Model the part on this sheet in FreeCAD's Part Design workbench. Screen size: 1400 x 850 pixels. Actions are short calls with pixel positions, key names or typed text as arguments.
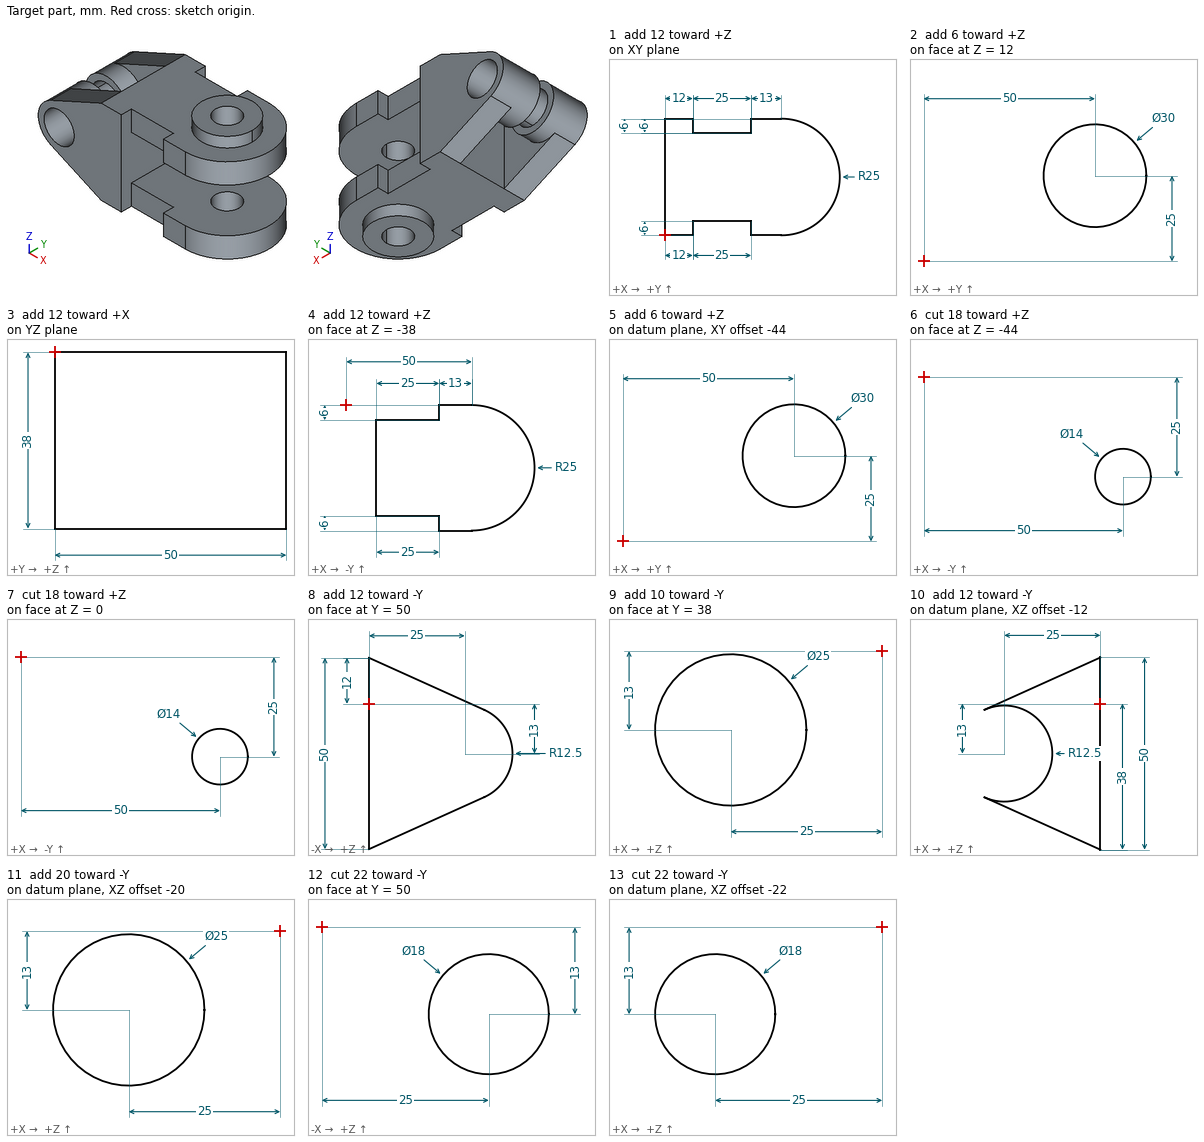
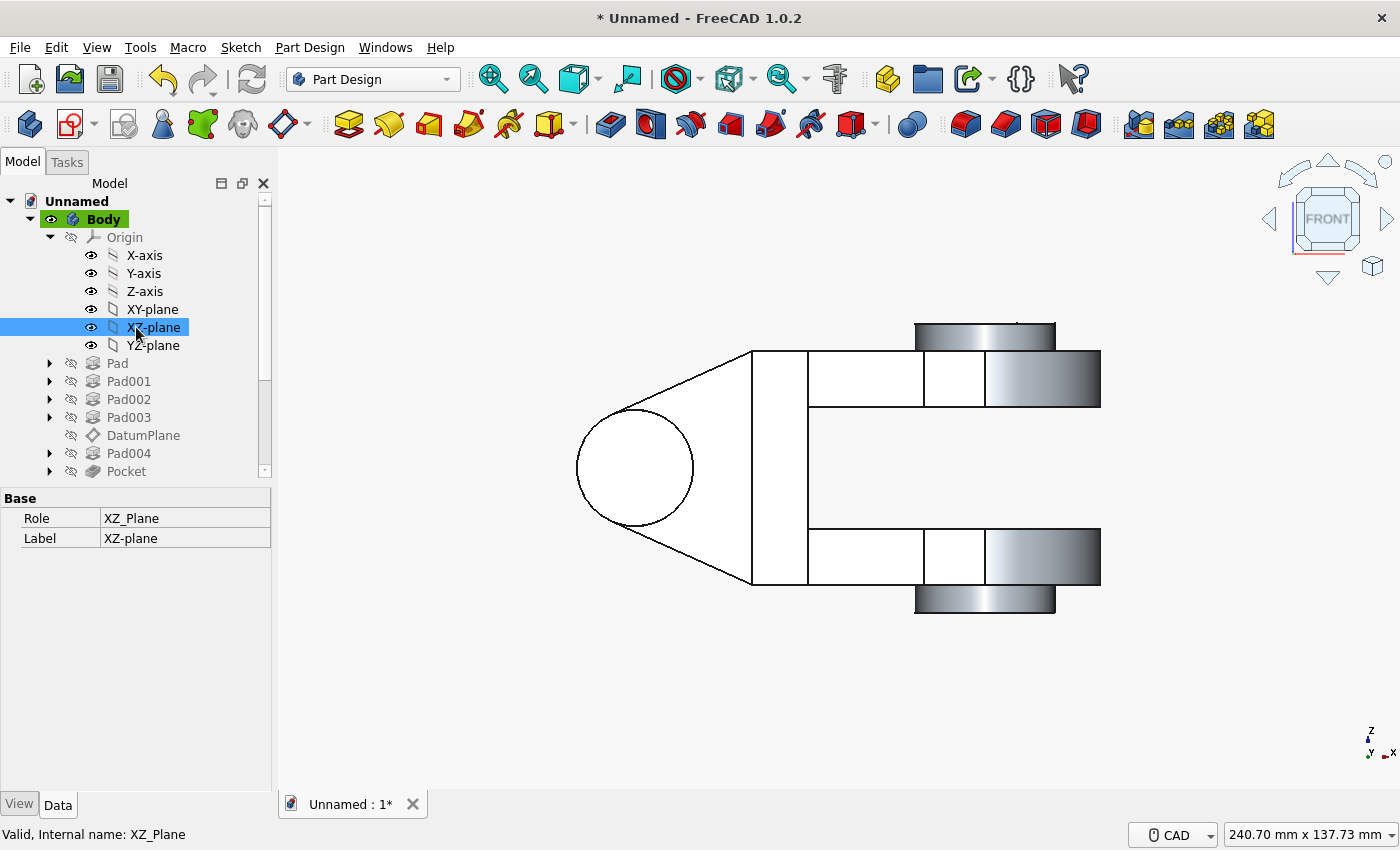
click(284, 124)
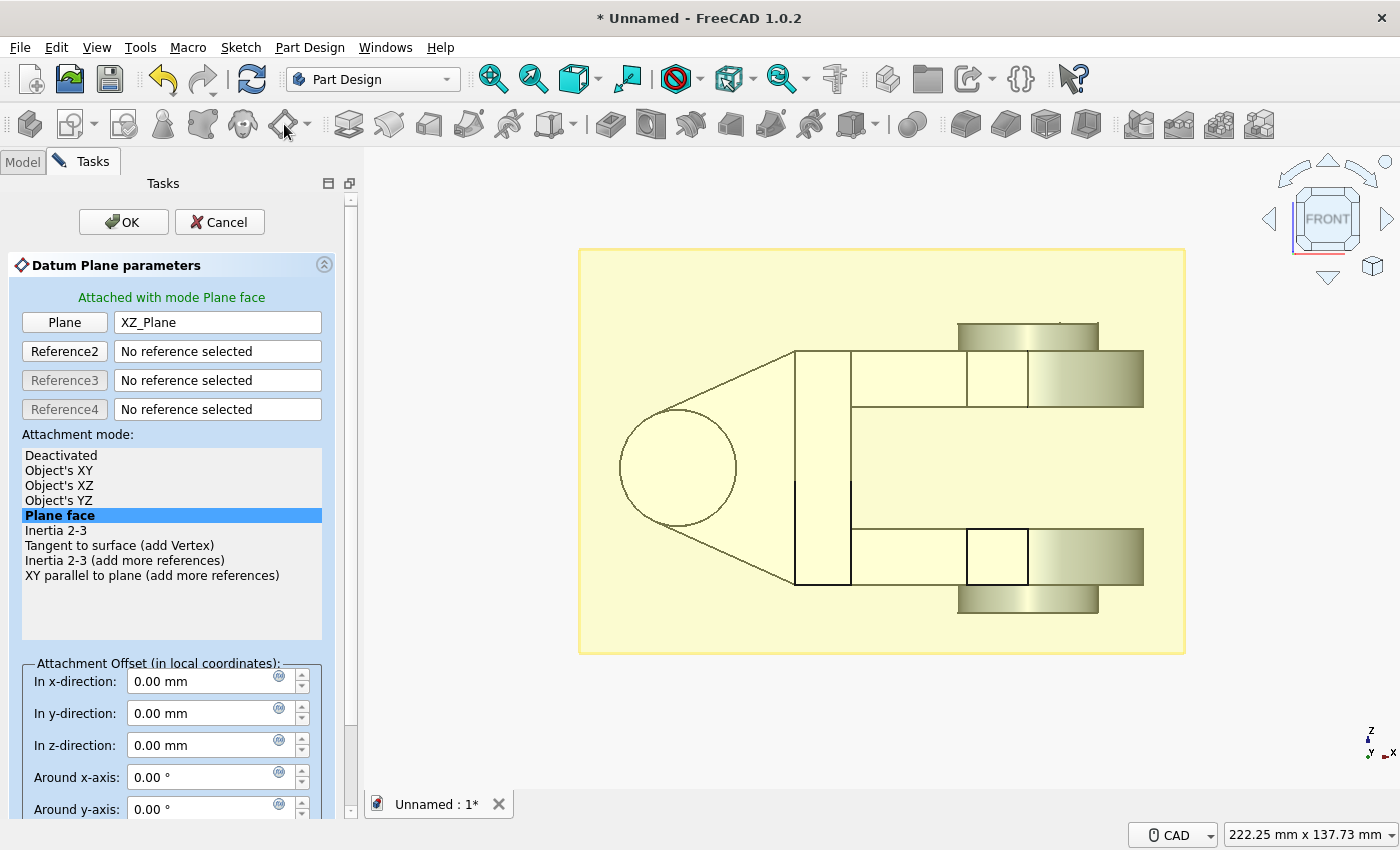
triple_click(210, 745)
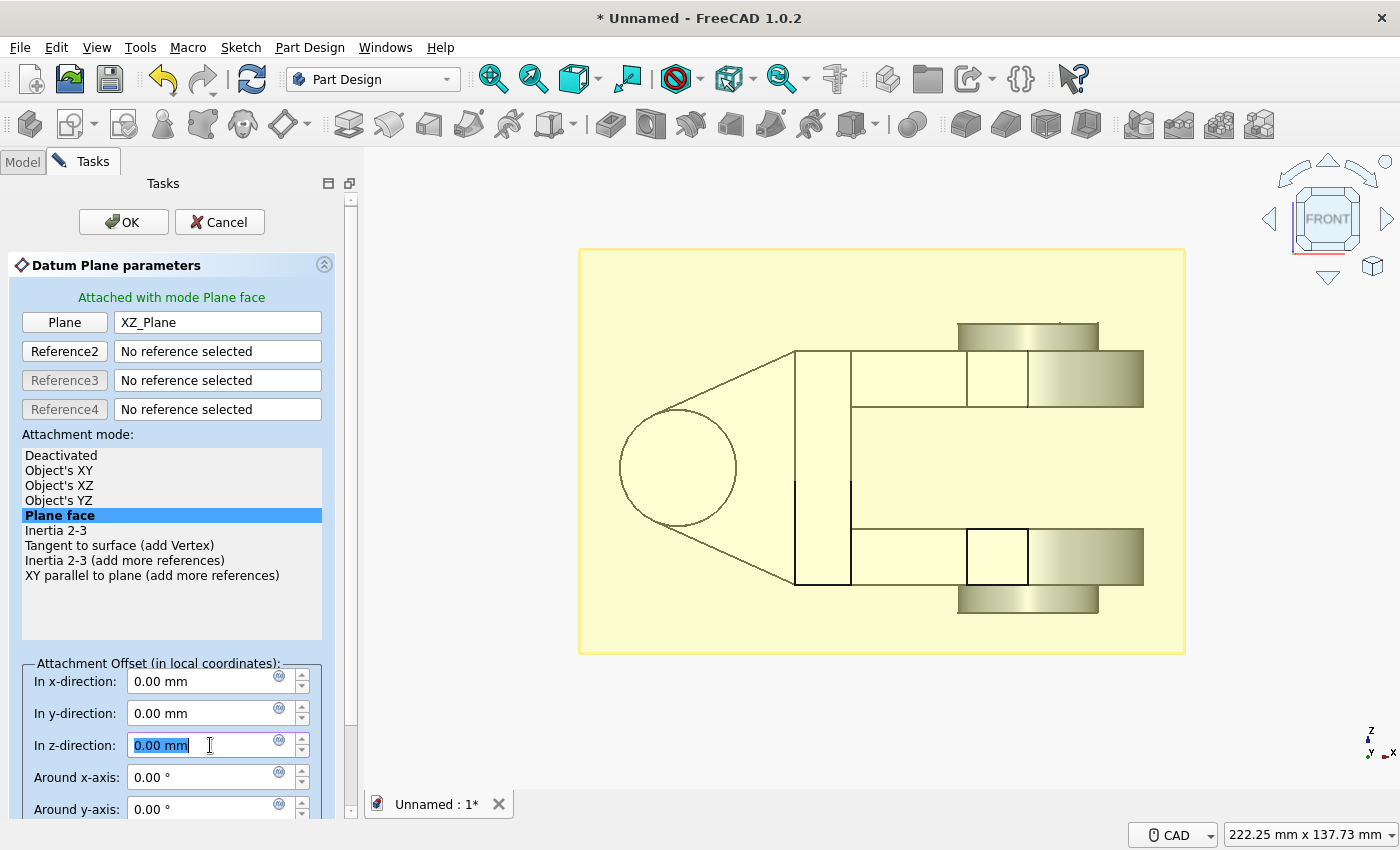
text(-12)
key(Tab)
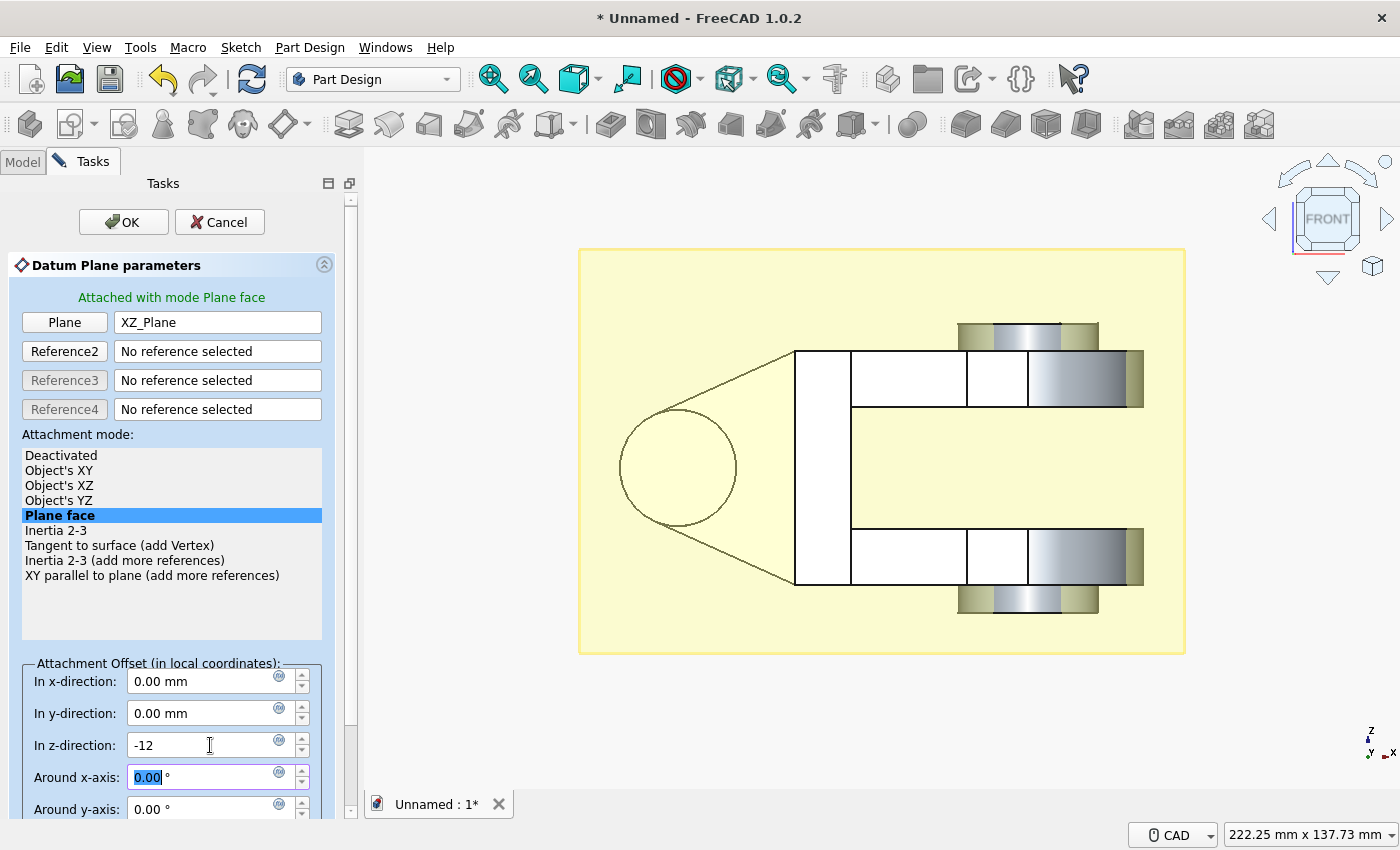
click(124, 222)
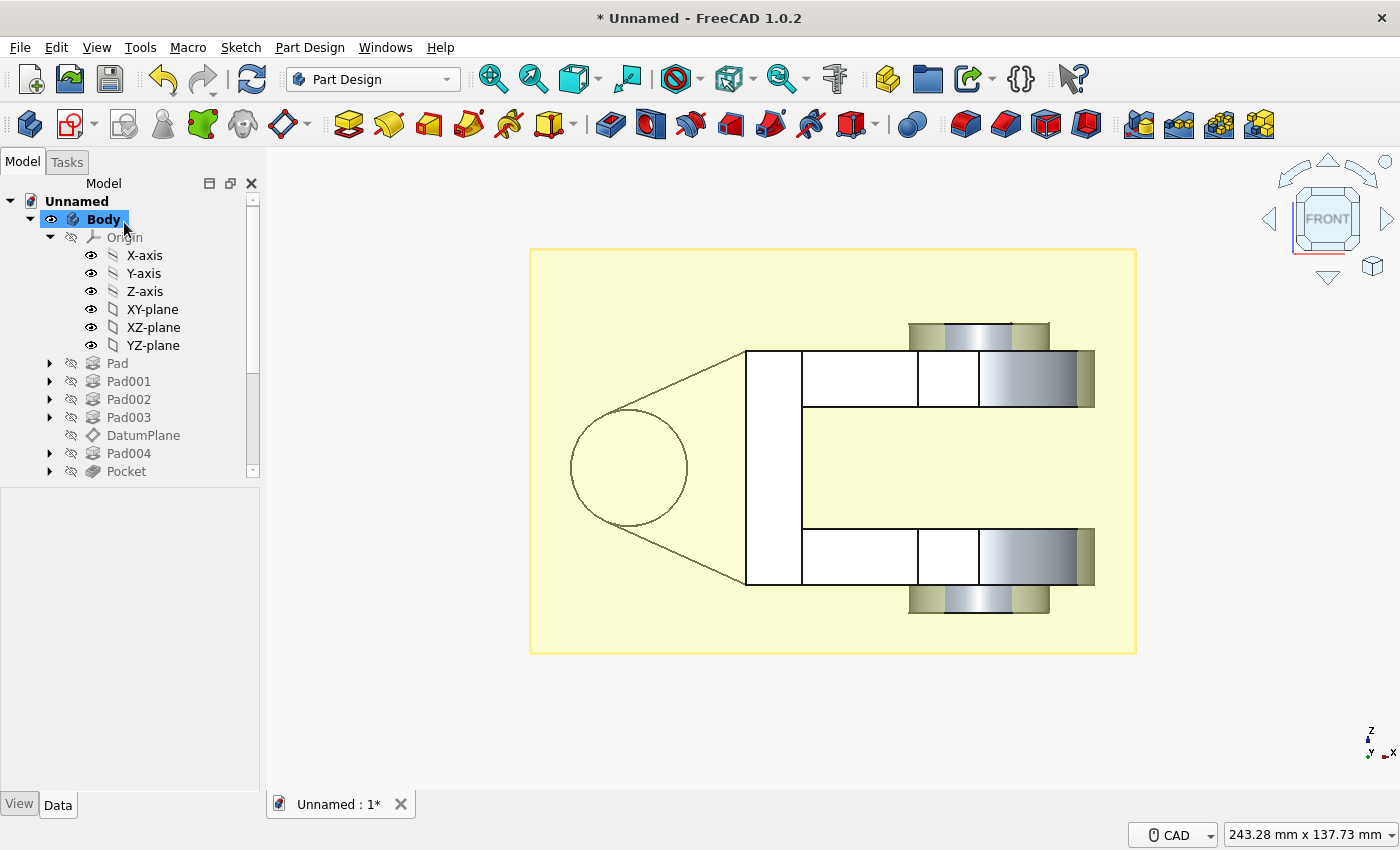
scroll(100, 341, down, 3)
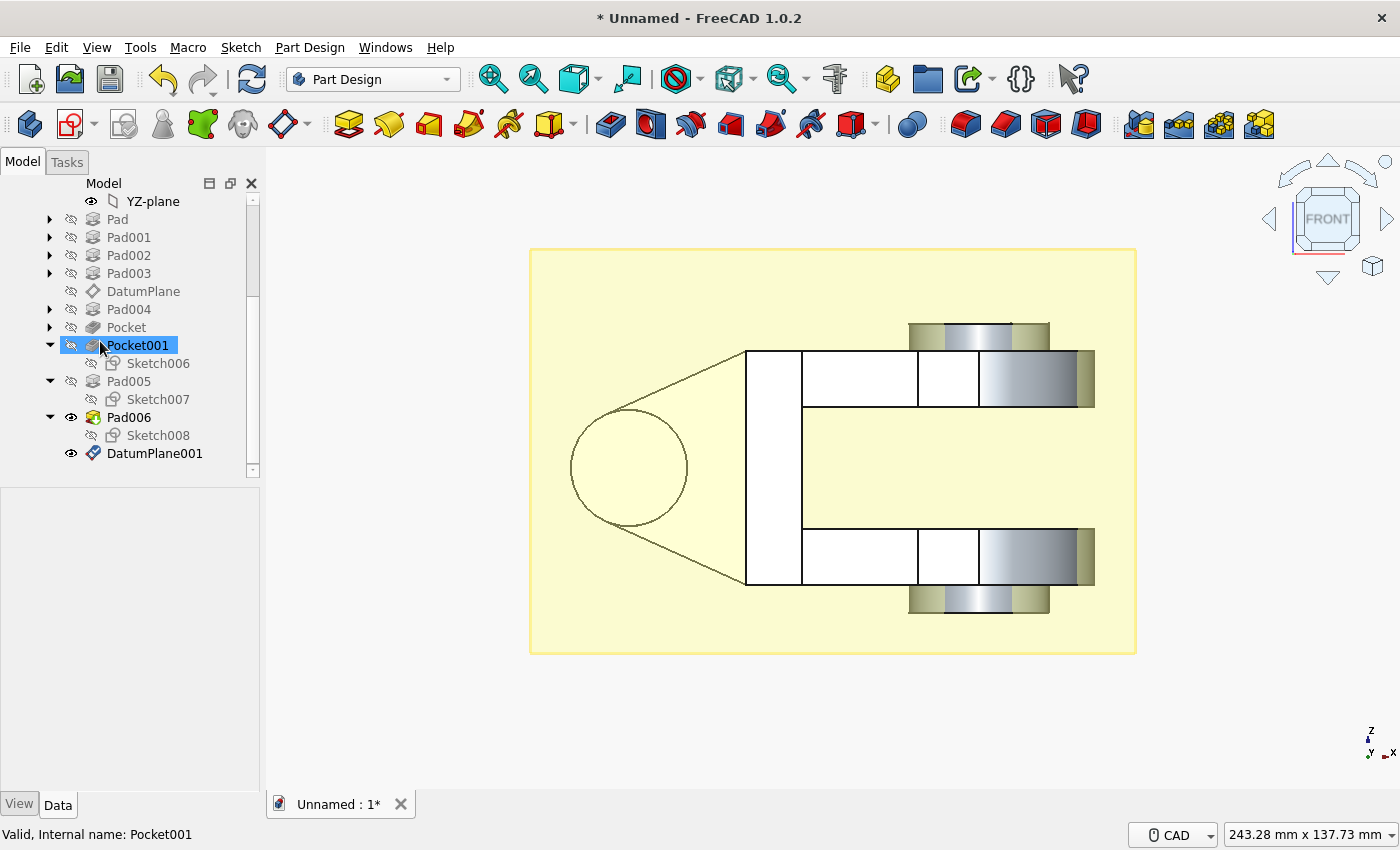
click(116, 453)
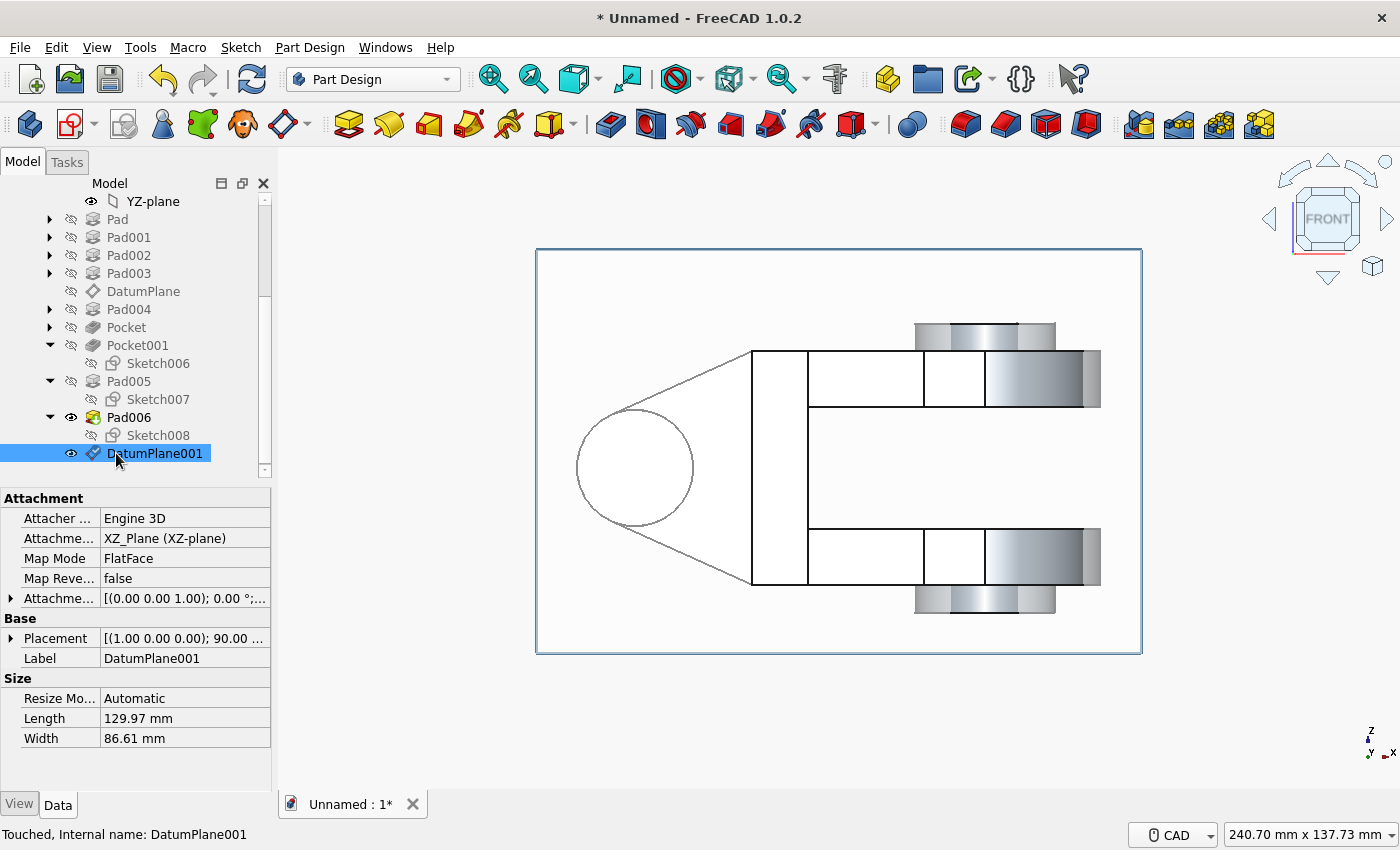
click(70, 124)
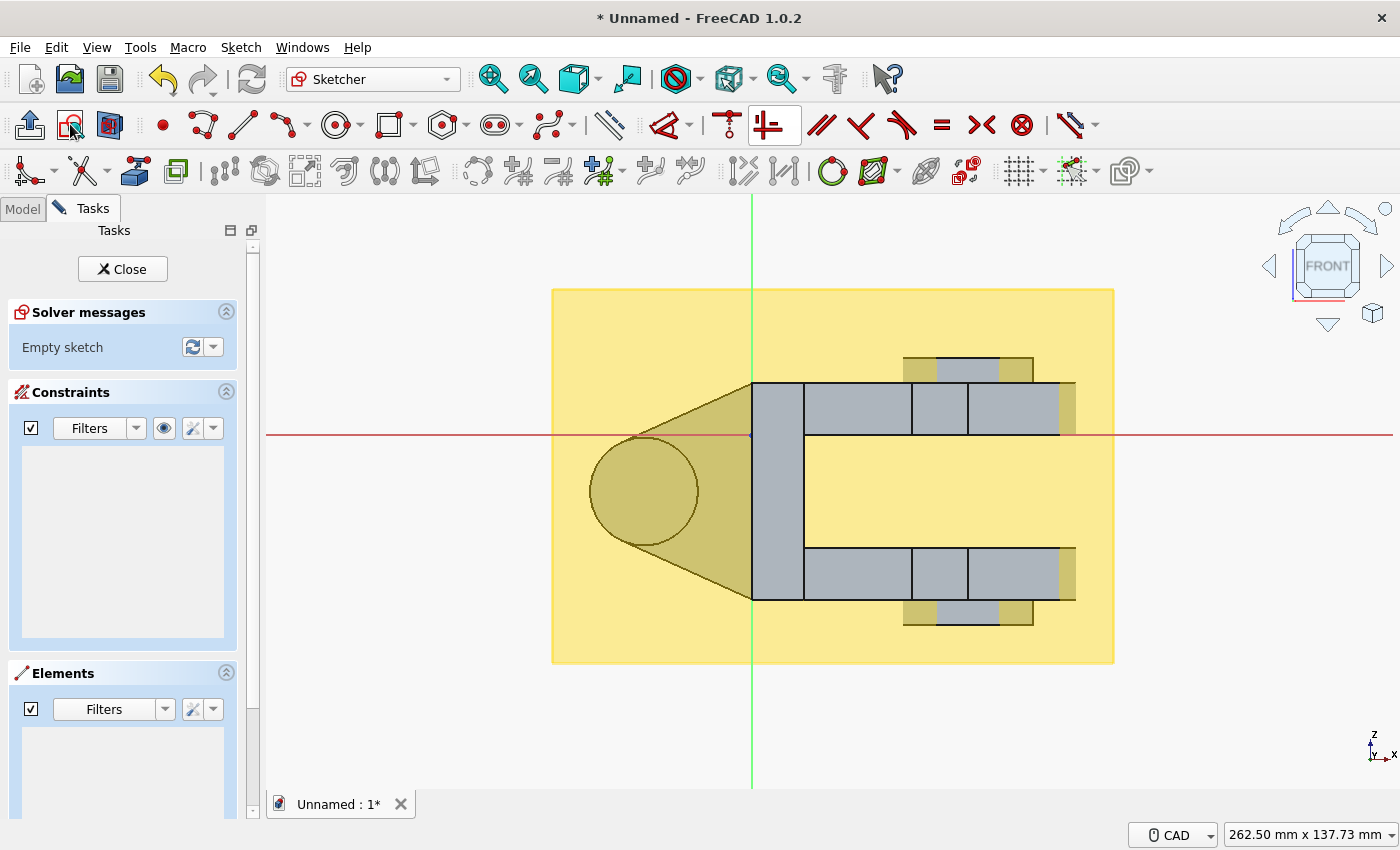
click(110, 126)